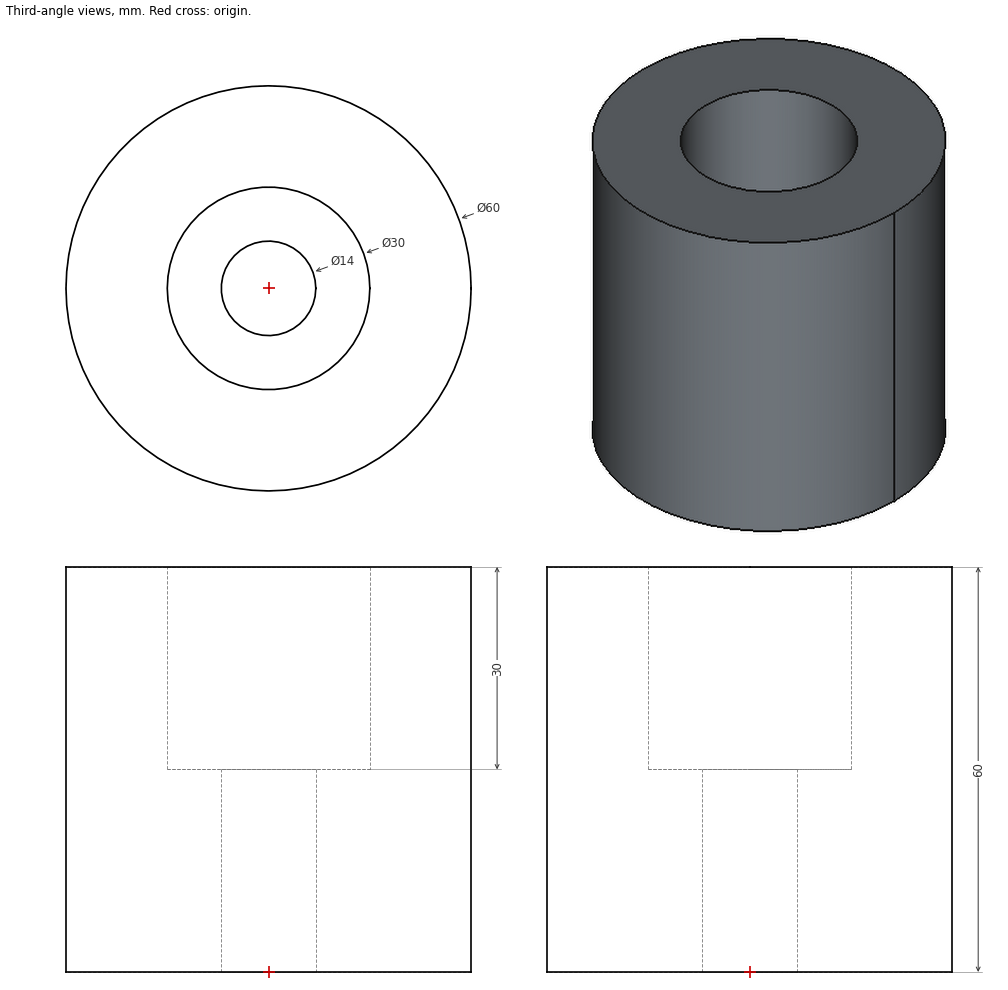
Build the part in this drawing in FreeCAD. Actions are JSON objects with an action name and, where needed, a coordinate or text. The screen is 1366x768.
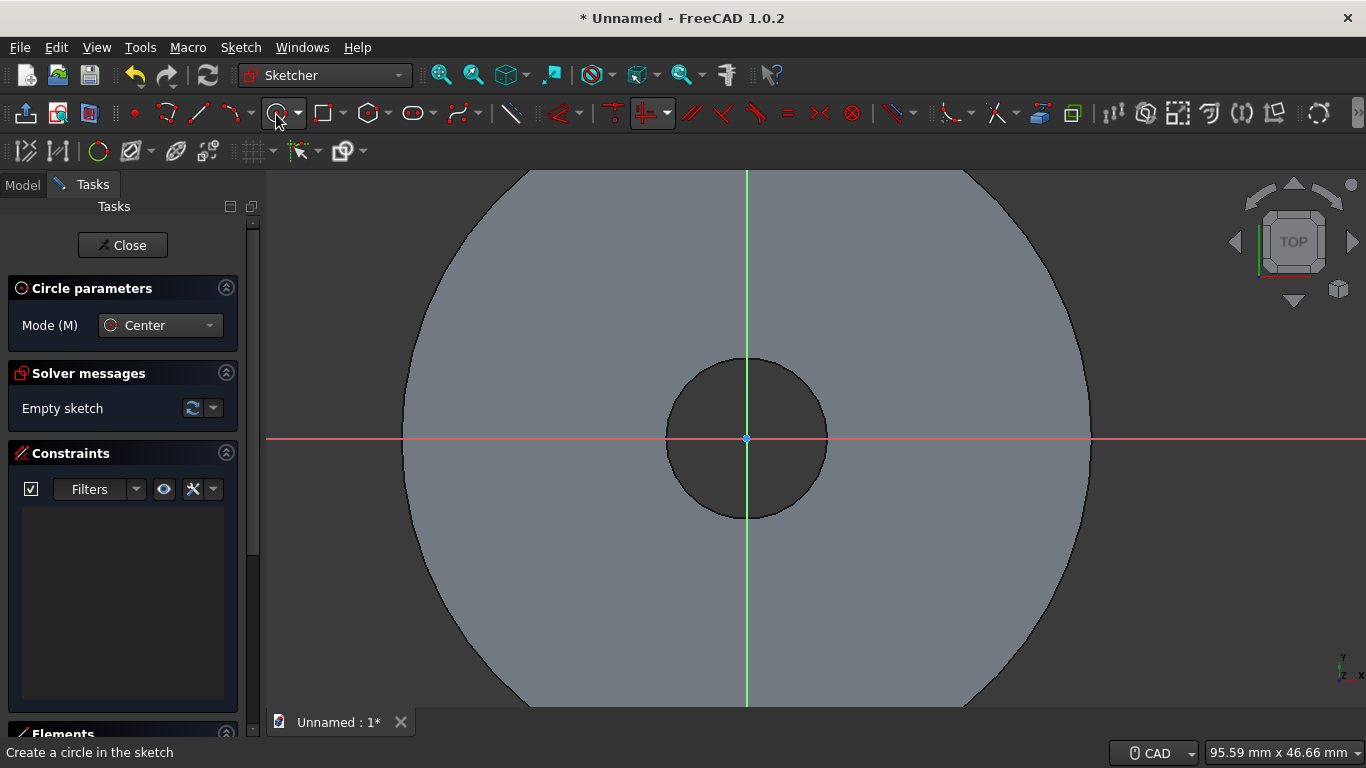
{"action": "left_click", "coordinate": [747, 438]}
{"action": "mouse_move", "coordinate": [869, 316]}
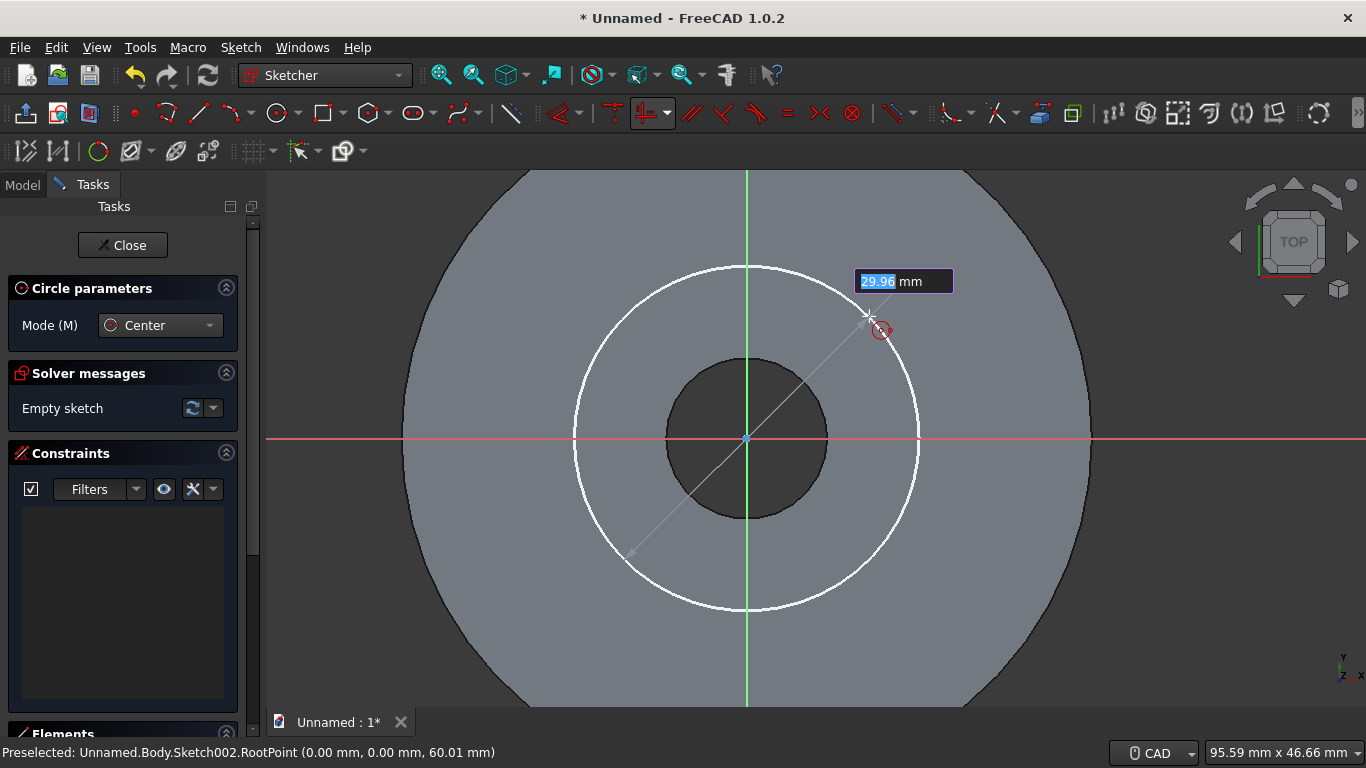
{"action": "type", "text": "30"}
{"action": "key", "text": "Return"}
{"action": "key", "text": "Escape"}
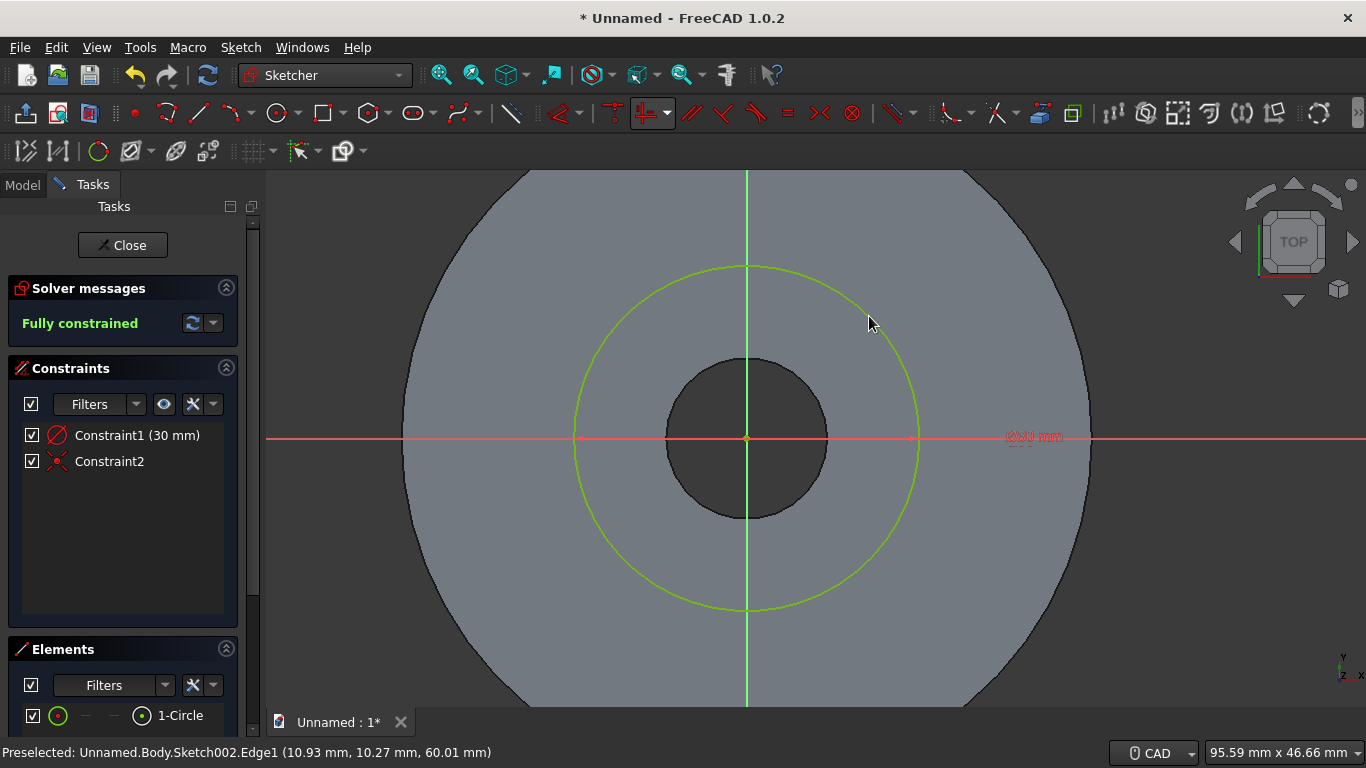
{"action": "left_click", "coordinate": [123, 245]}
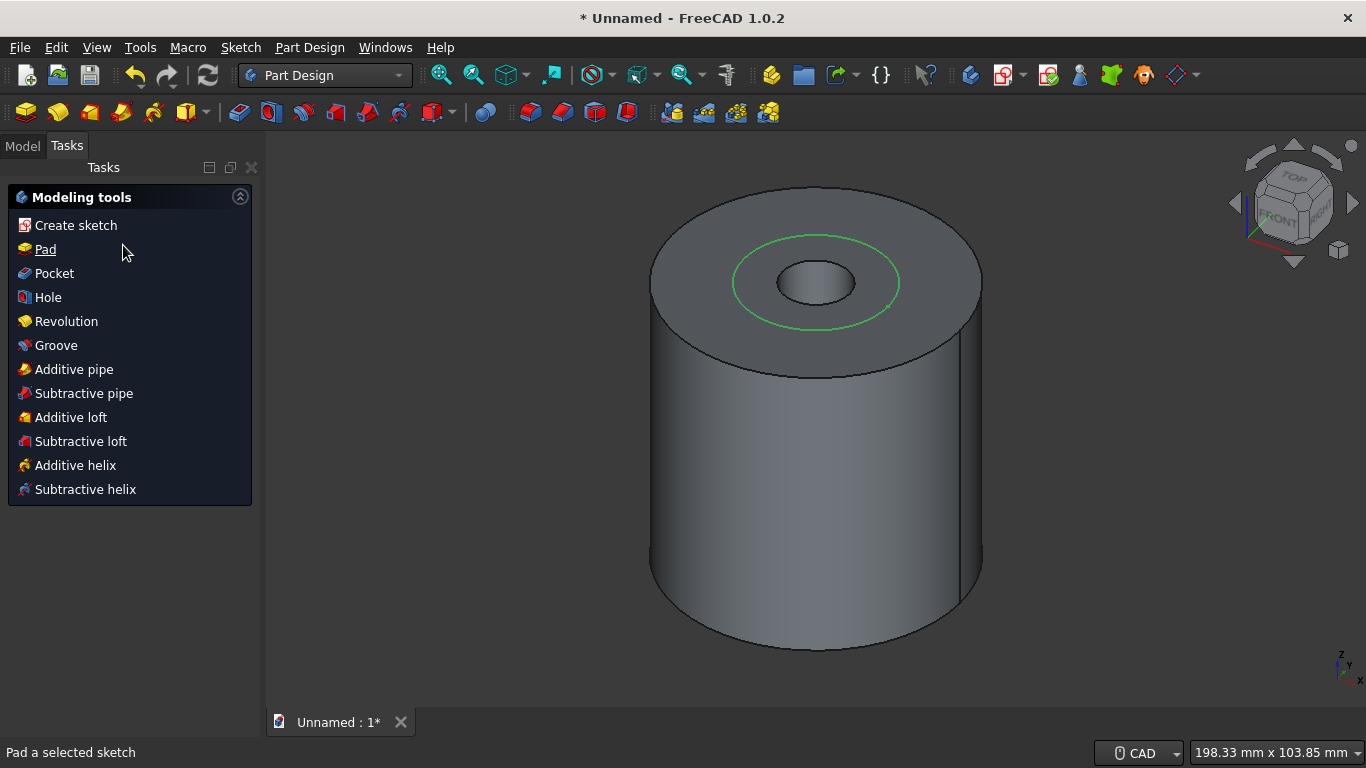
{"action": "left_click", "coordinate": [240, 112]}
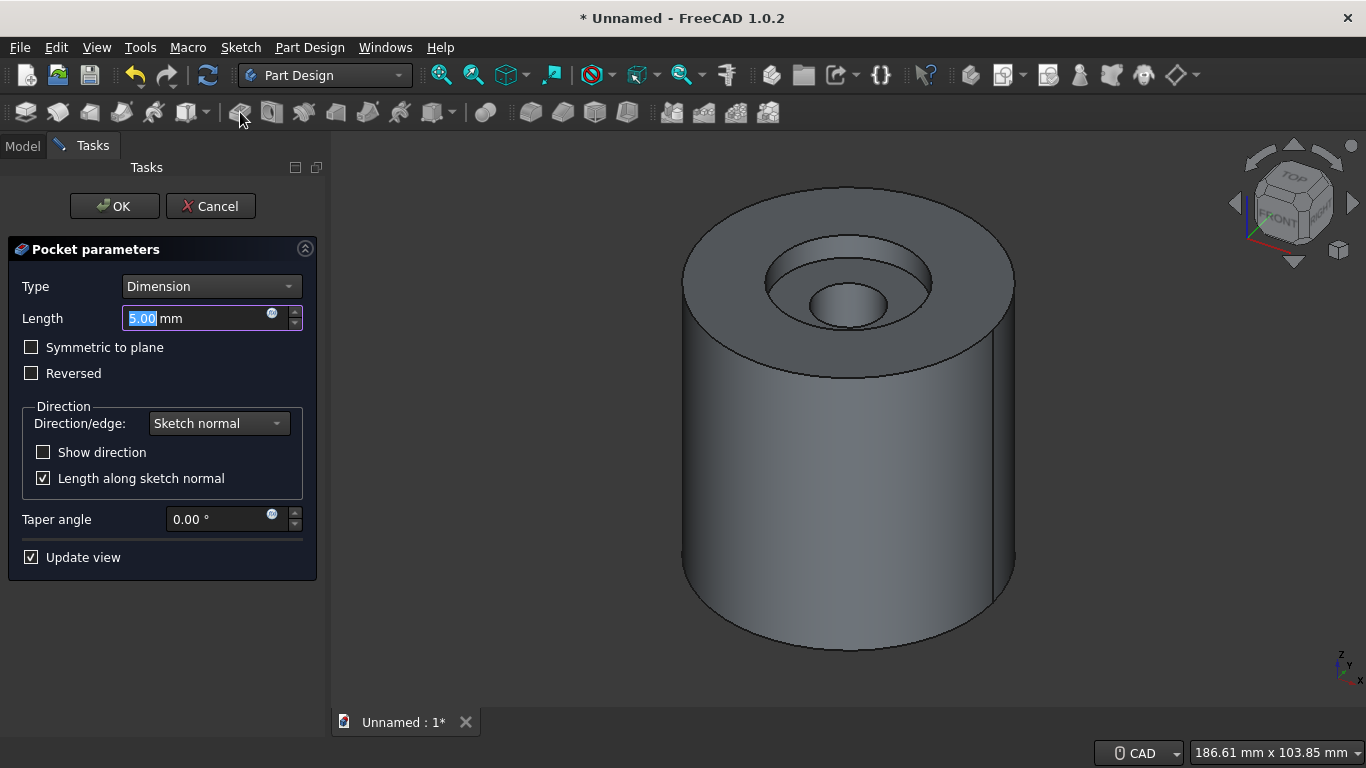
{"action": "type", "text": "30"}
{"action": "key", "text": "Tab"}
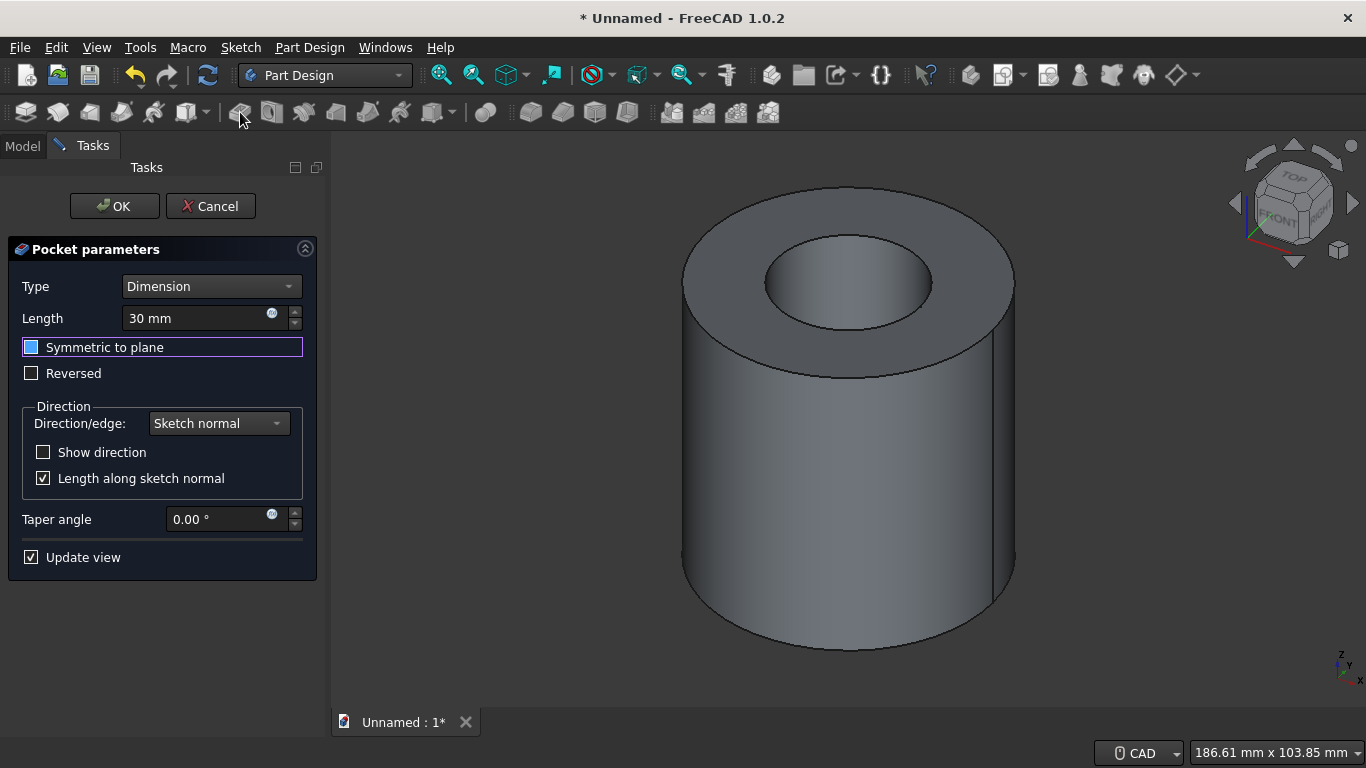
{"action": "left_click", "coordinate": [115, 206]}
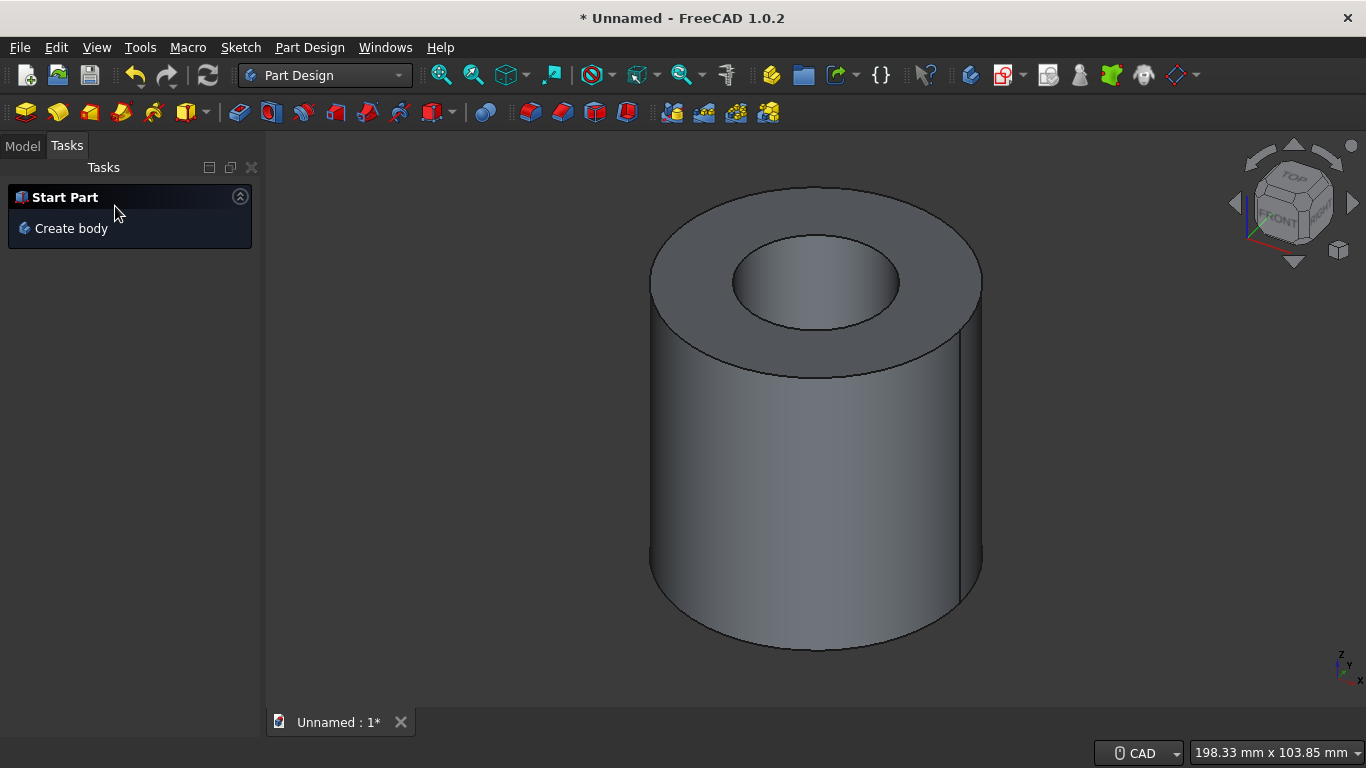
{"action": "key", "text": "0"}